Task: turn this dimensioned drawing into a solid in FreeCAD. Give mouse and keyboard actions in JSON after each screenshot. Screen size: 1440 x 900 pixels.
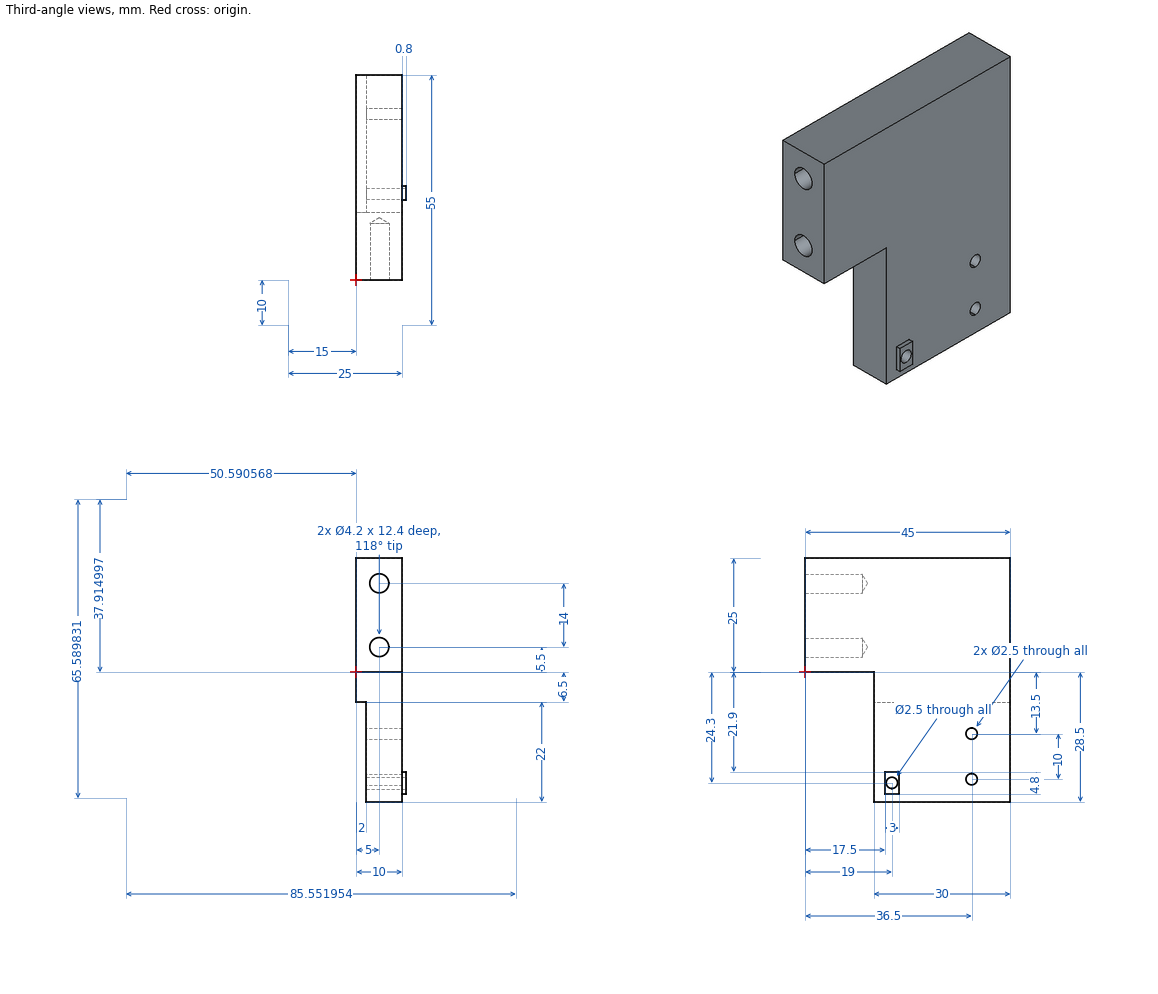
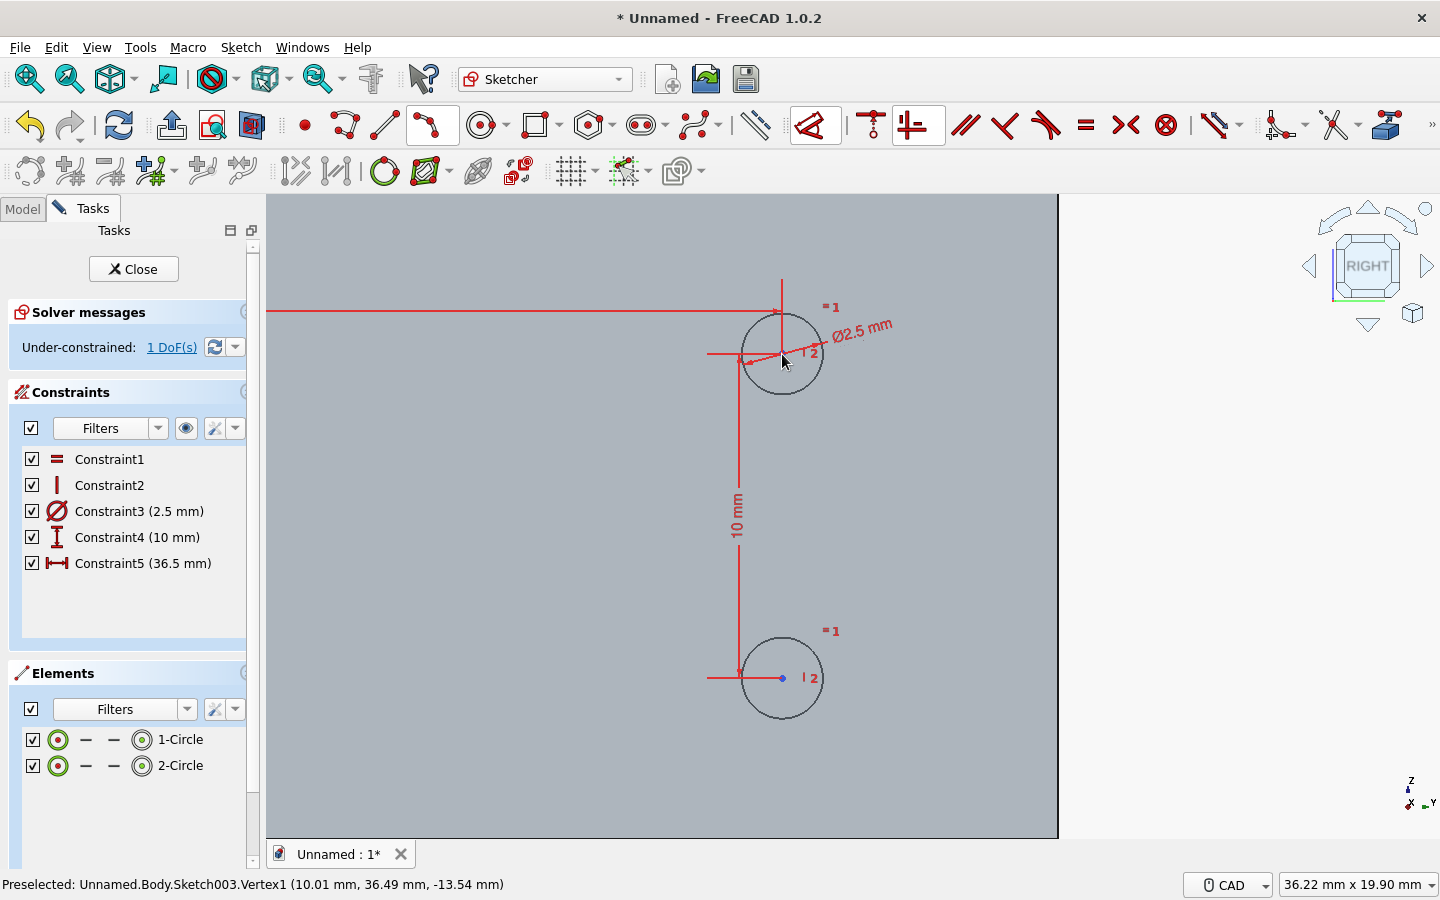
{"action": "left_click", "coordinate": [782, 354]}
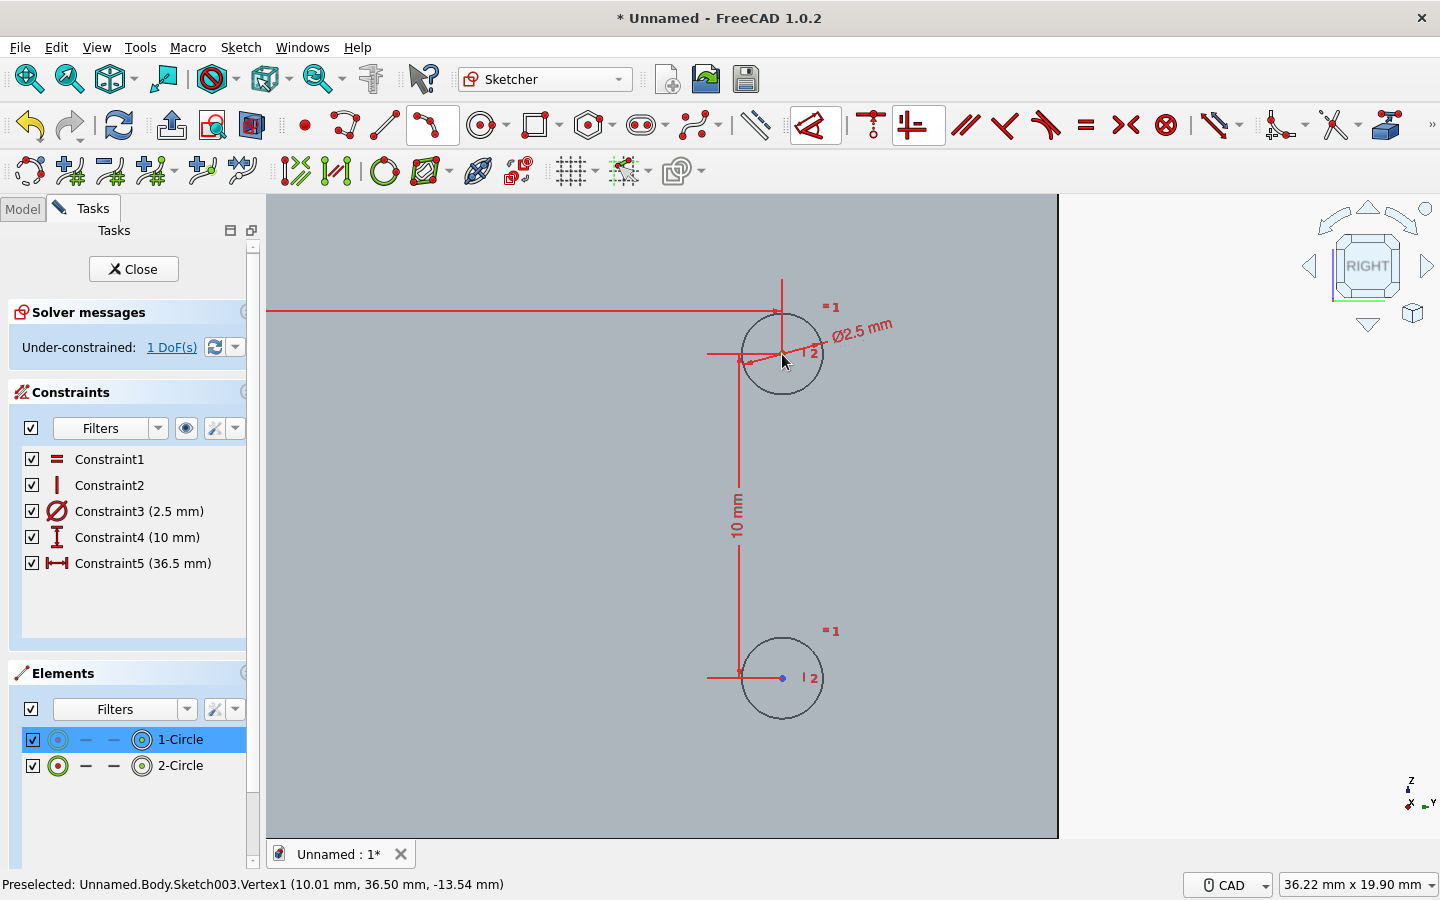
{"action": "key", "text": "i"}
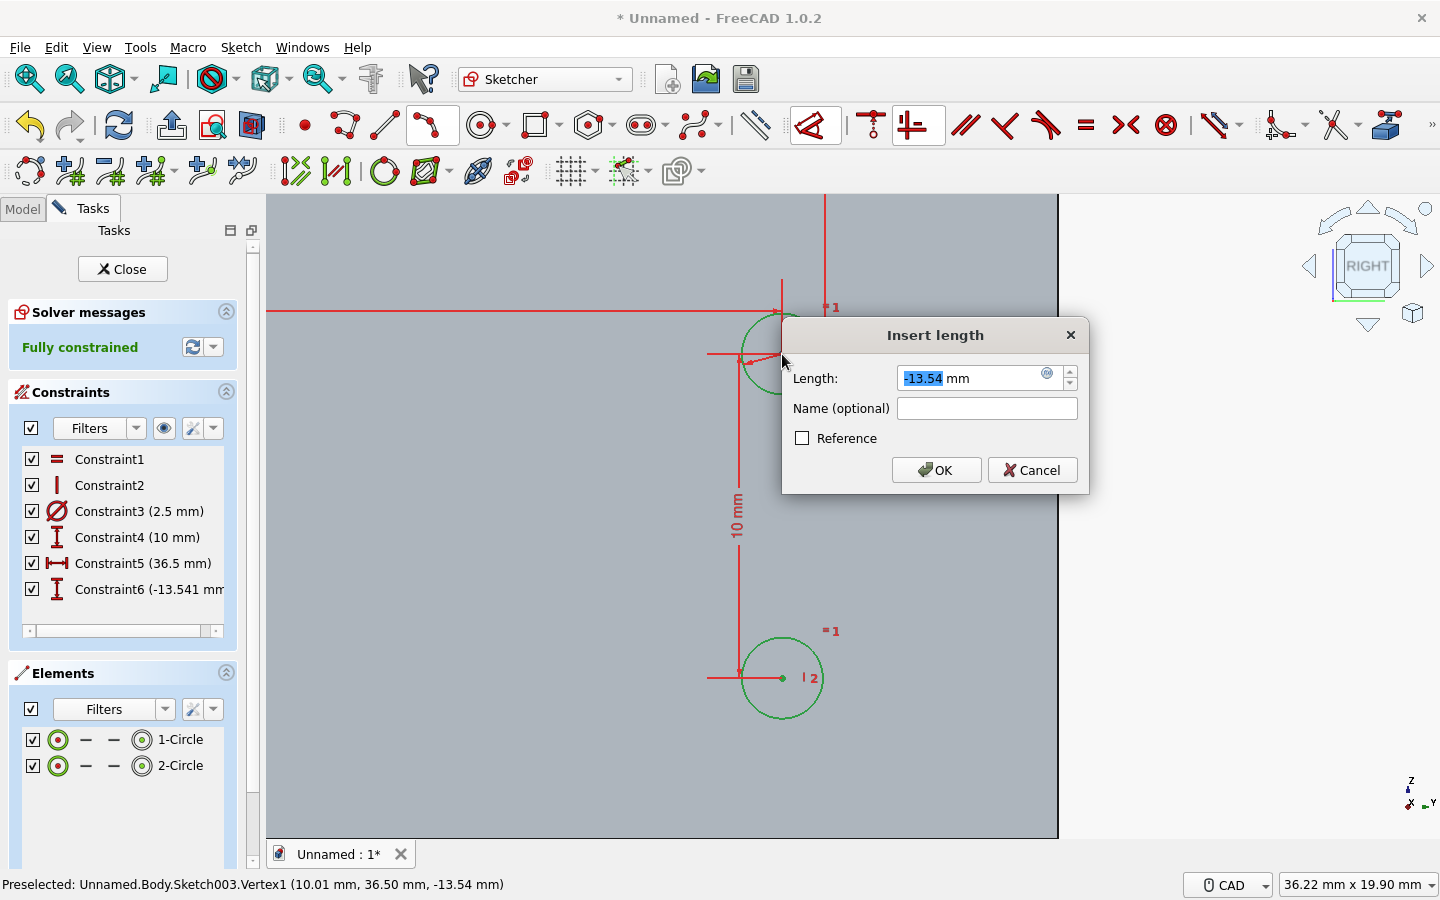
{"action": "type", "text": "-13.5"}
{"action": "key", "text": "Return"}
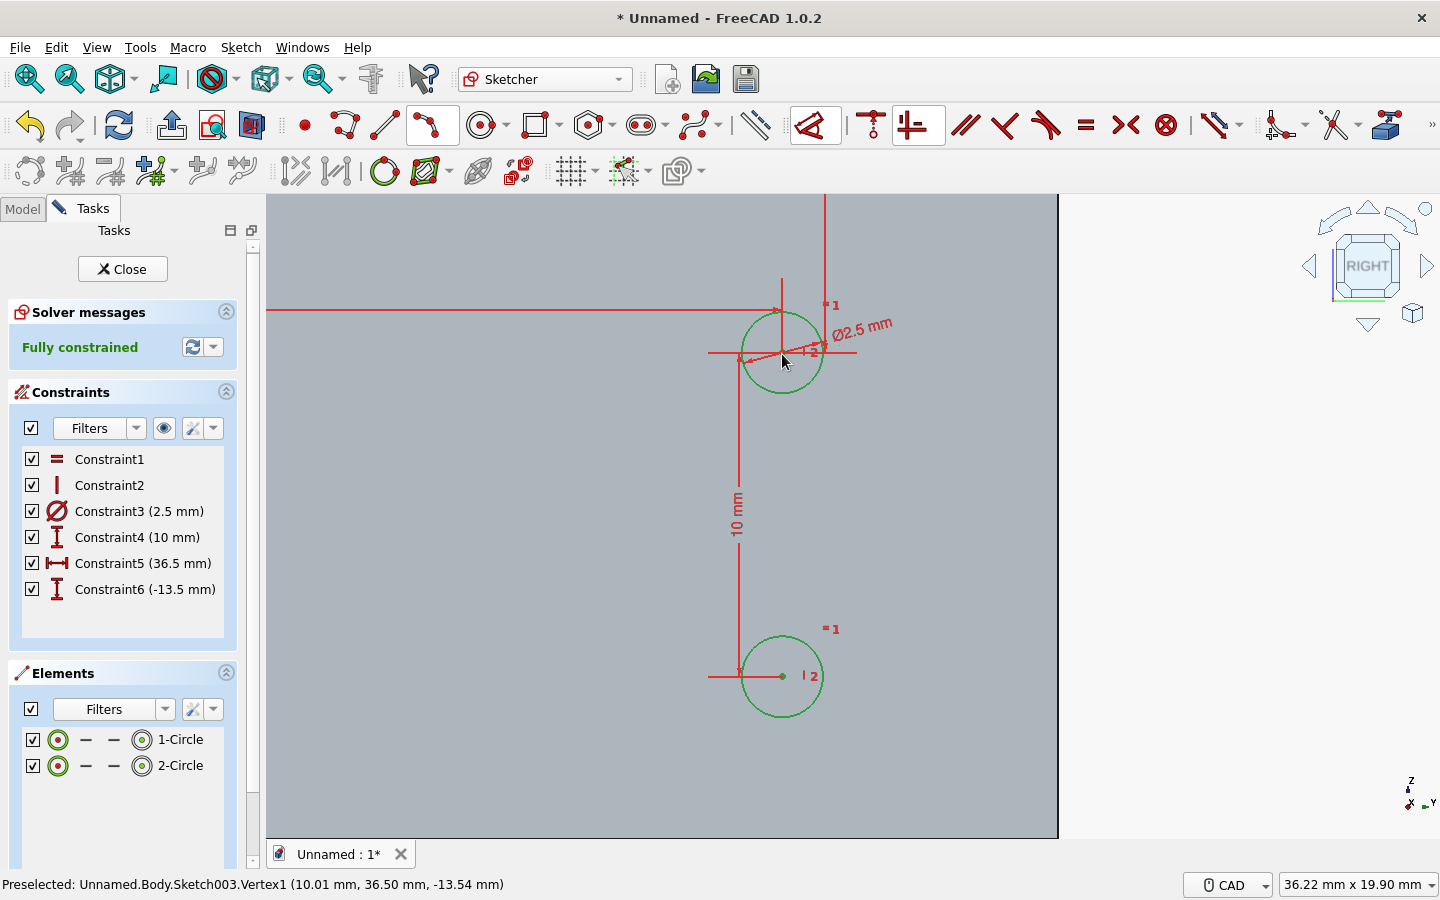
{"action": "left_click", "coordinate": [123, 269]}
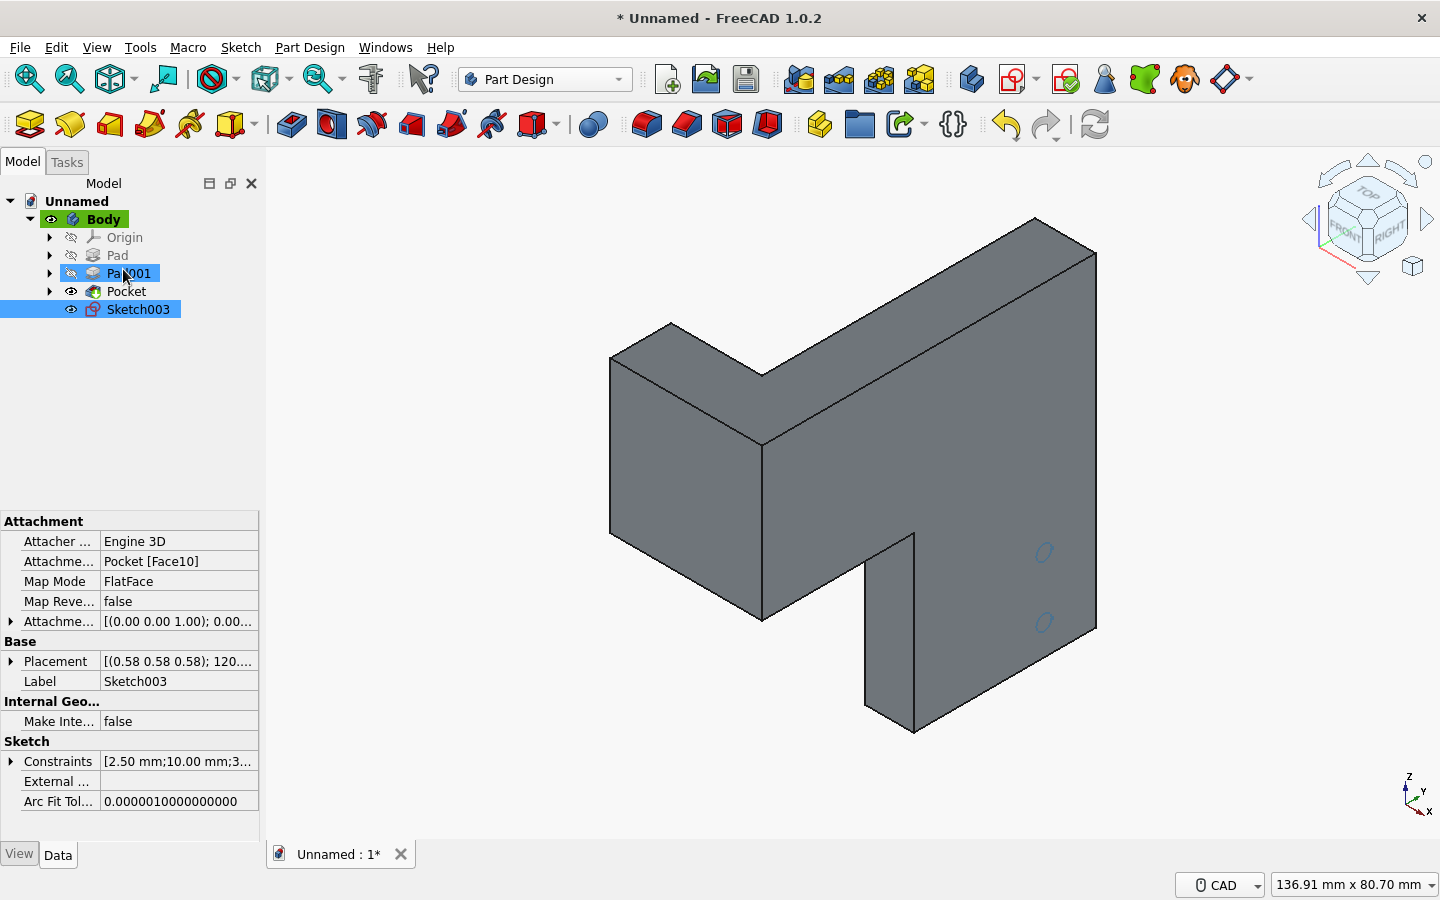
{"action": "left_click", "coordinate": [332, 124]}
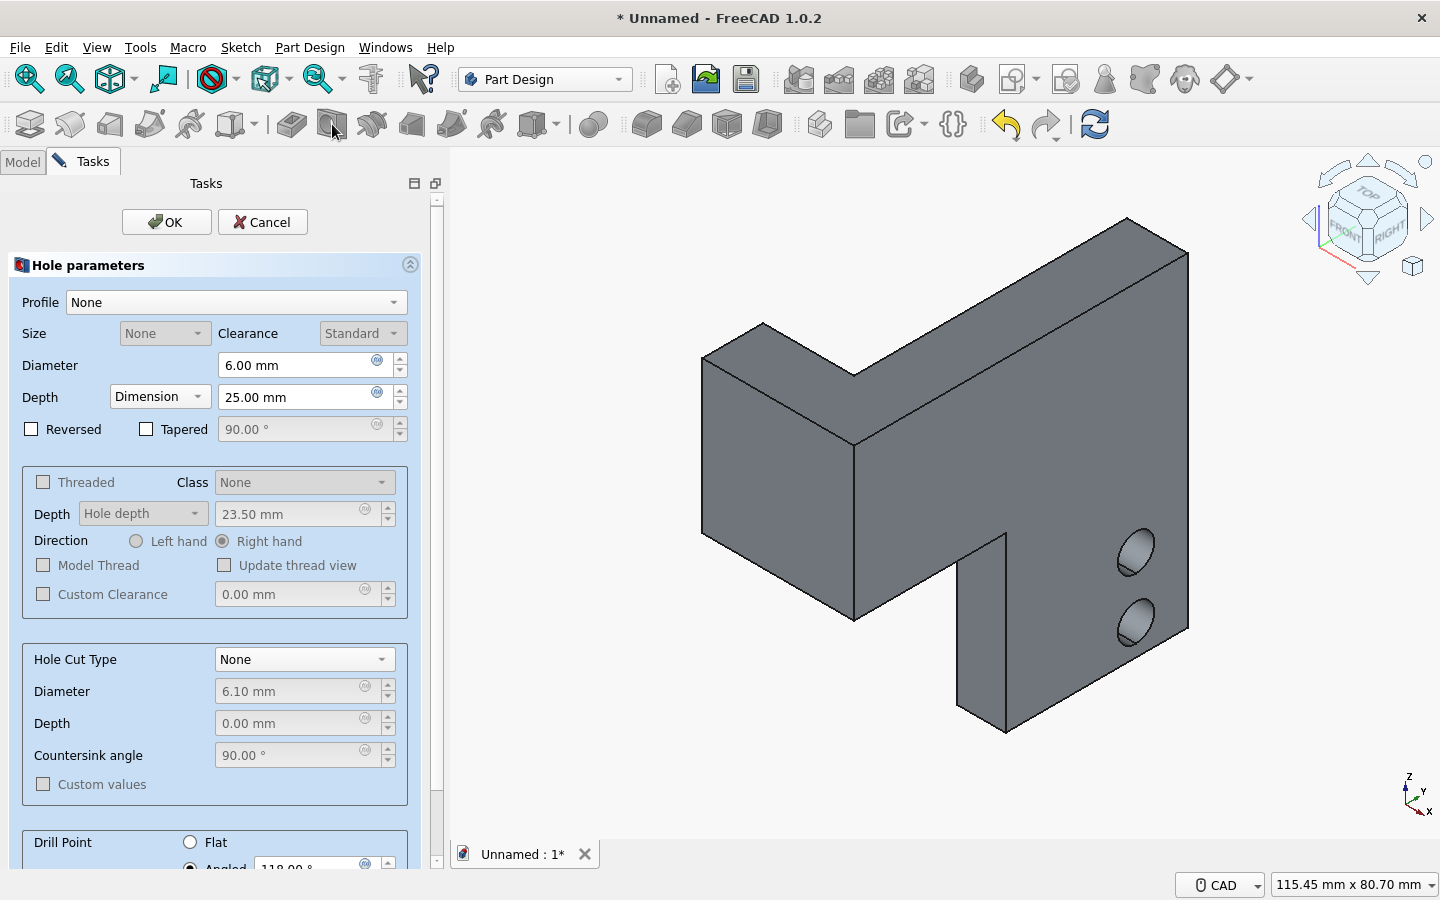
{"action": "triple_click", "coordinate": [305, 365]}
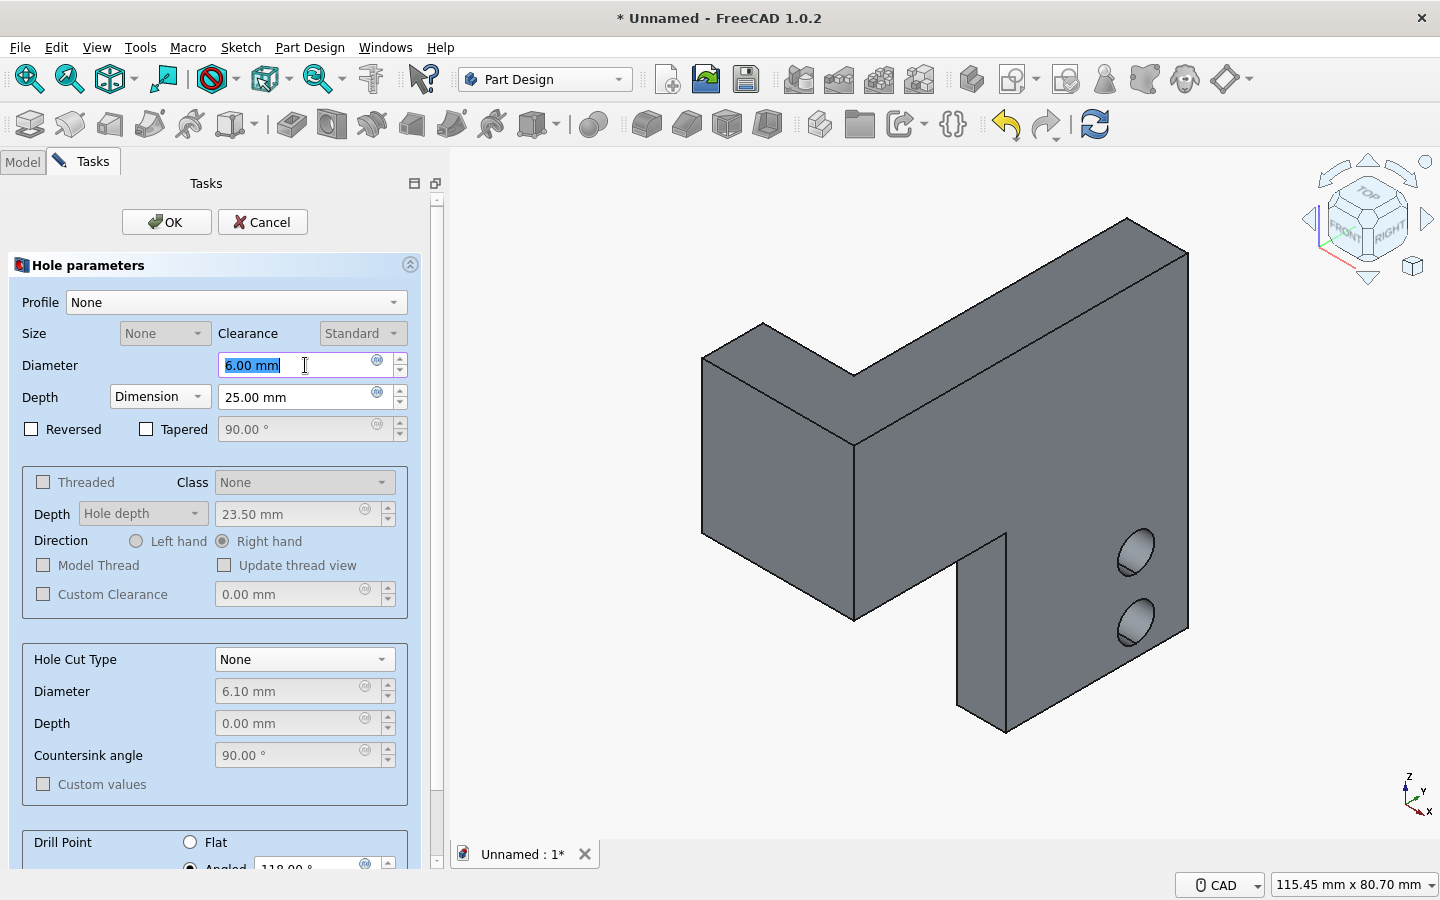
{"action": "type", "text": "2.5"}
{"action": "key", "text": "Tab"}